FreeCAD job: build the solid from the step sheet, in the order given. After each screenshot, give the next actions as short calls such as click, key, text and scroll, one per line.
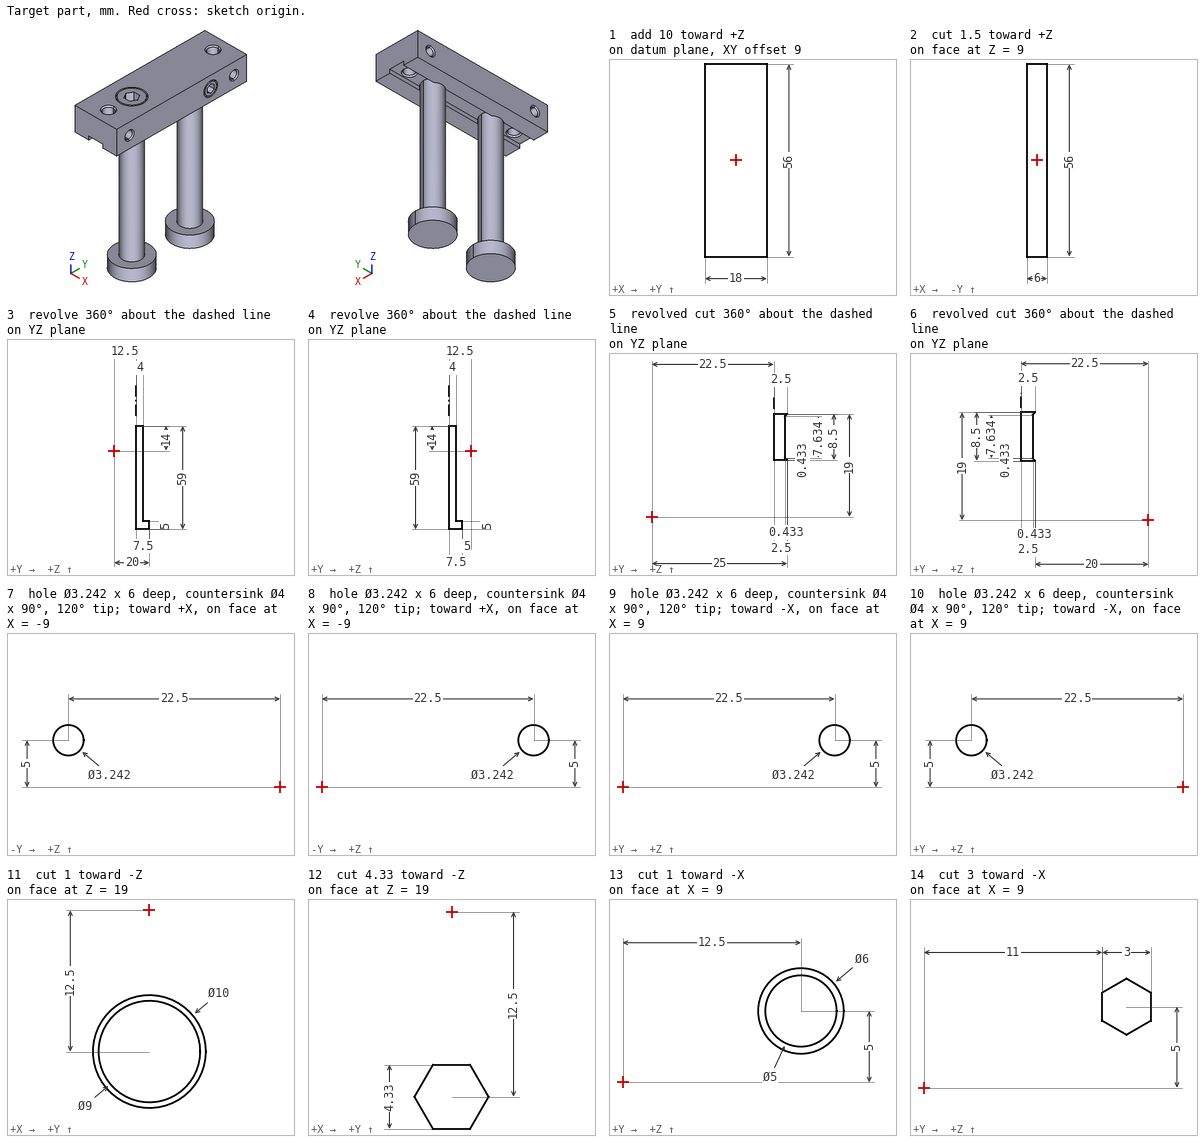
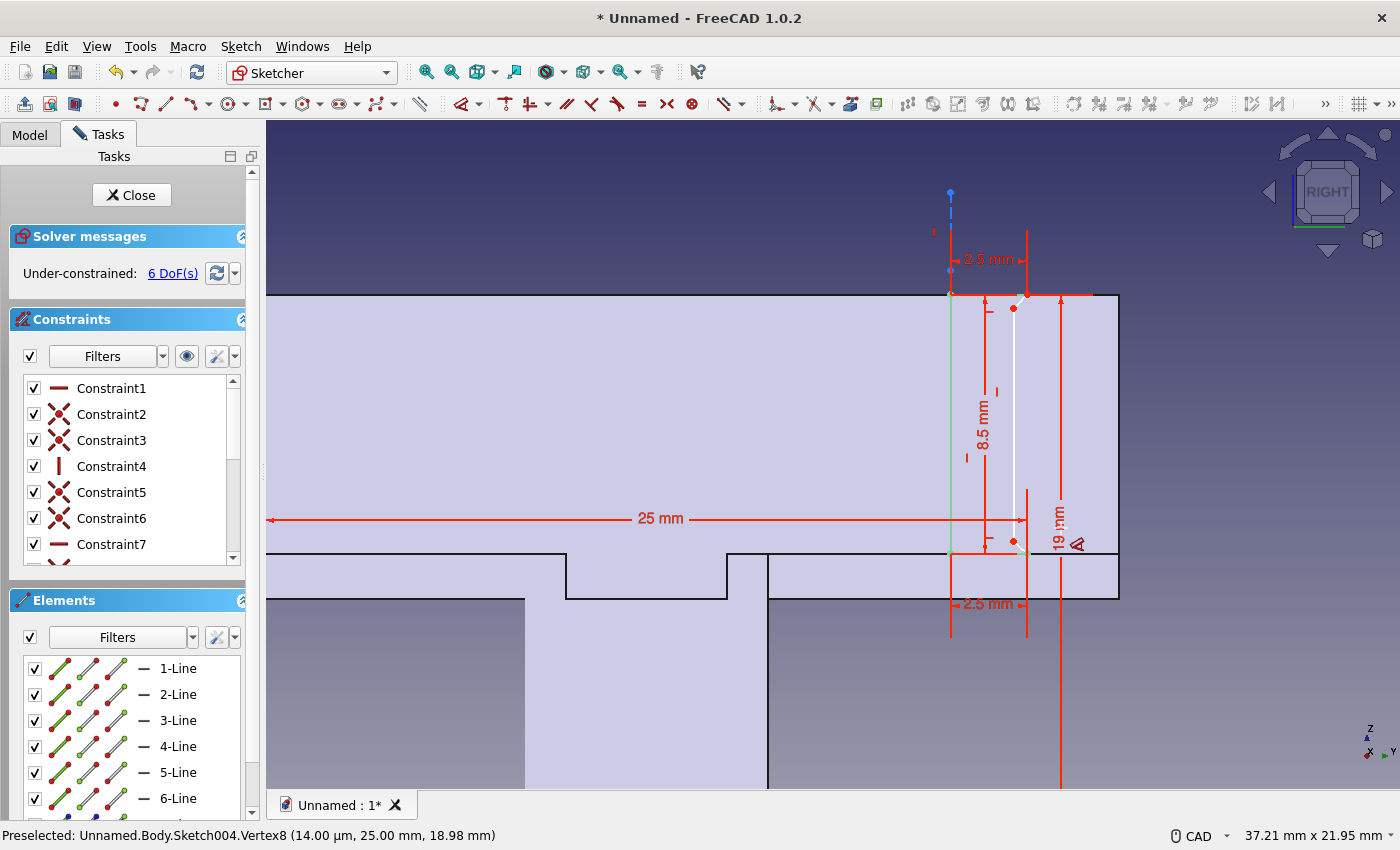
click(1014, 472)
click(1048, 371)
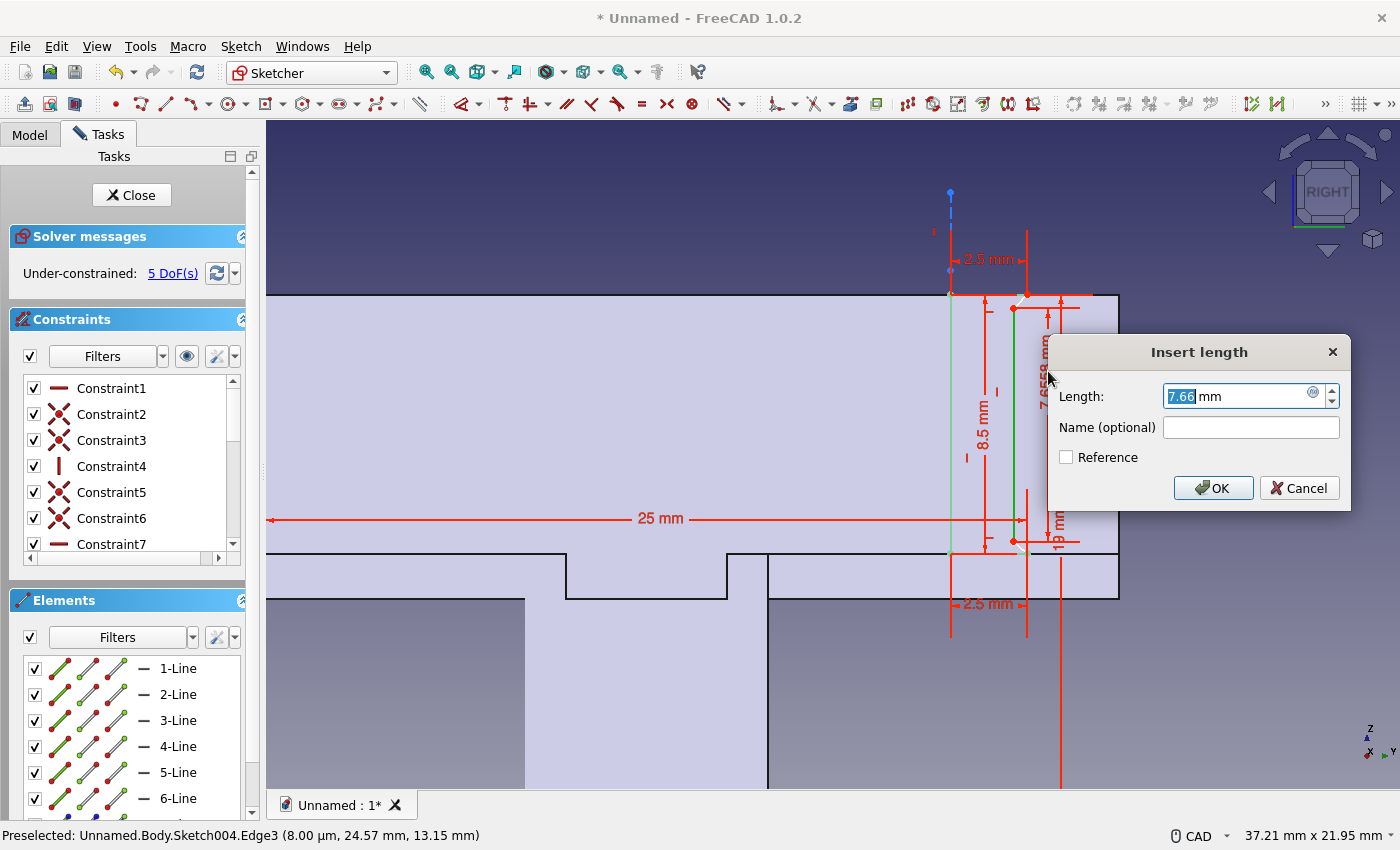
text(7.634)
key(Return)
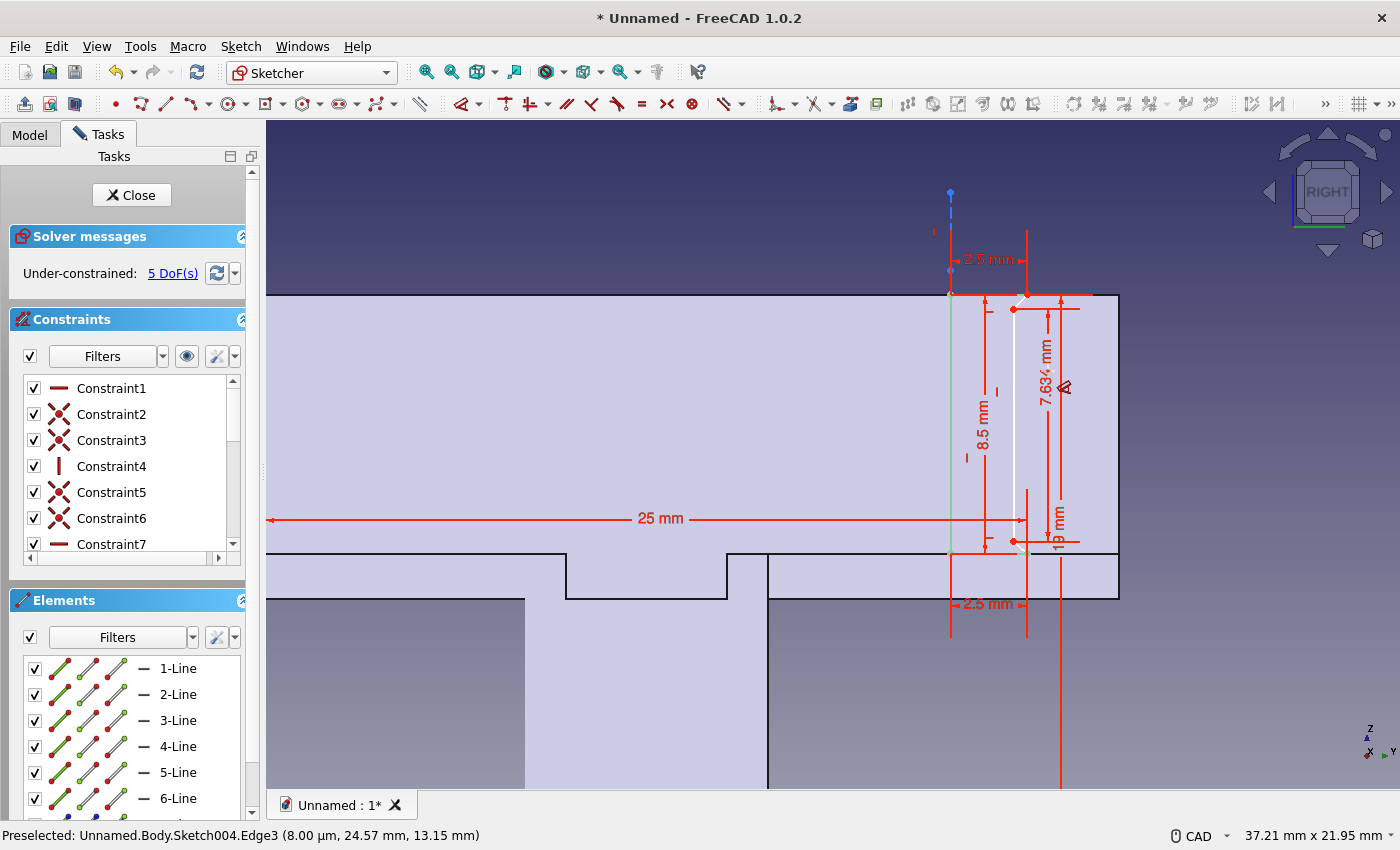
click(951, 271)
click(622, 237)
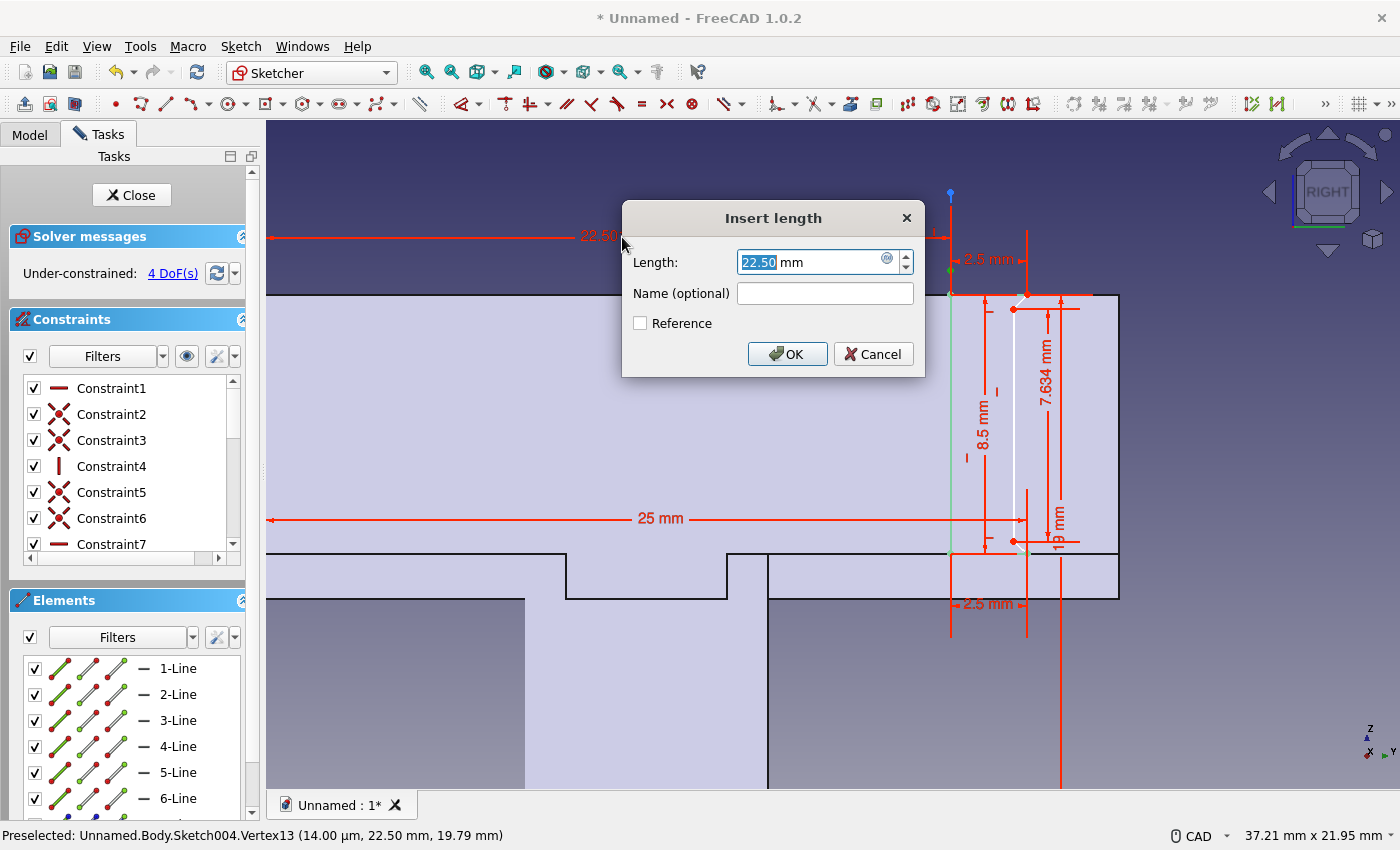
text(22.5)
key(Return)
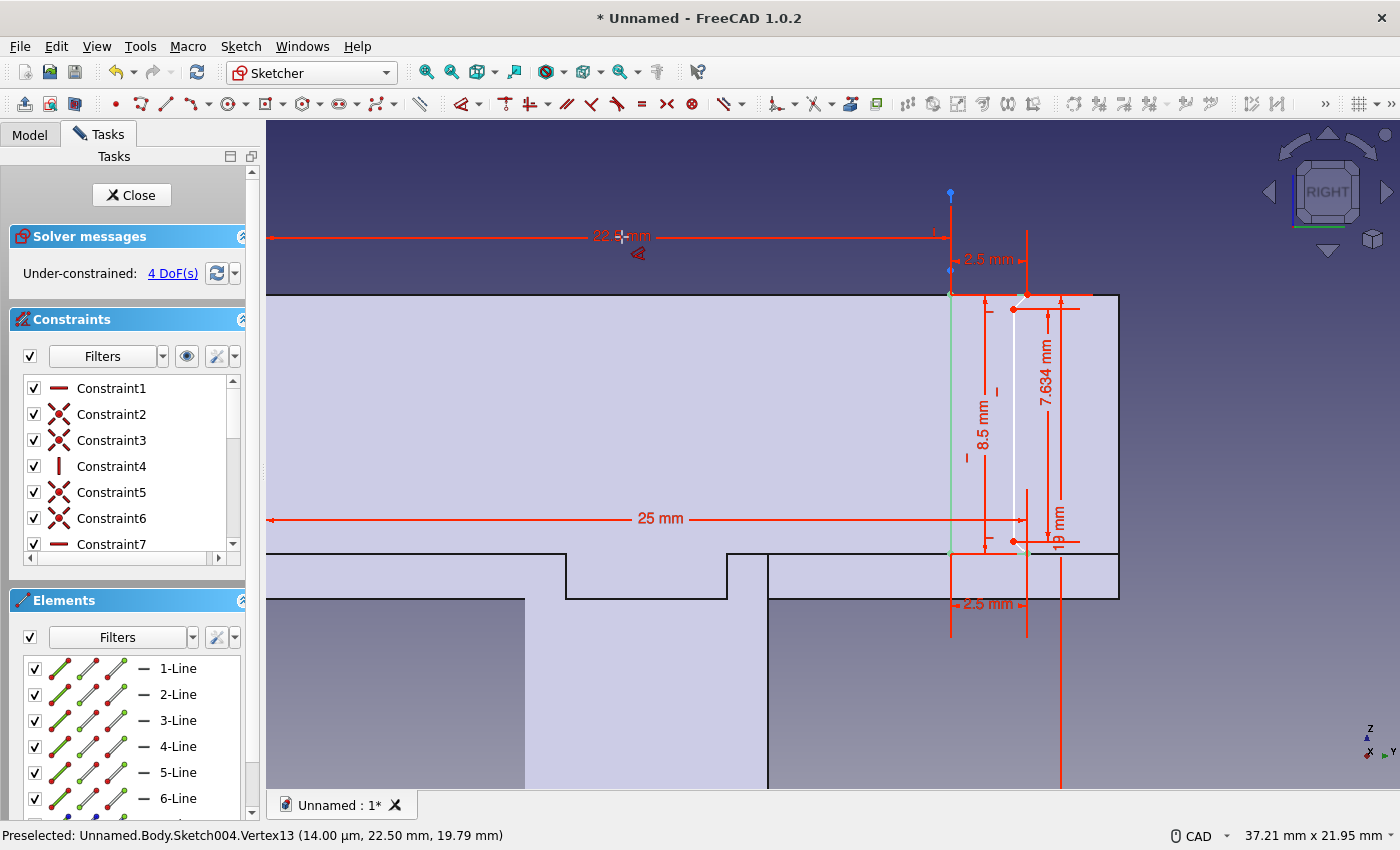
scroll(1019, 547, up, 6)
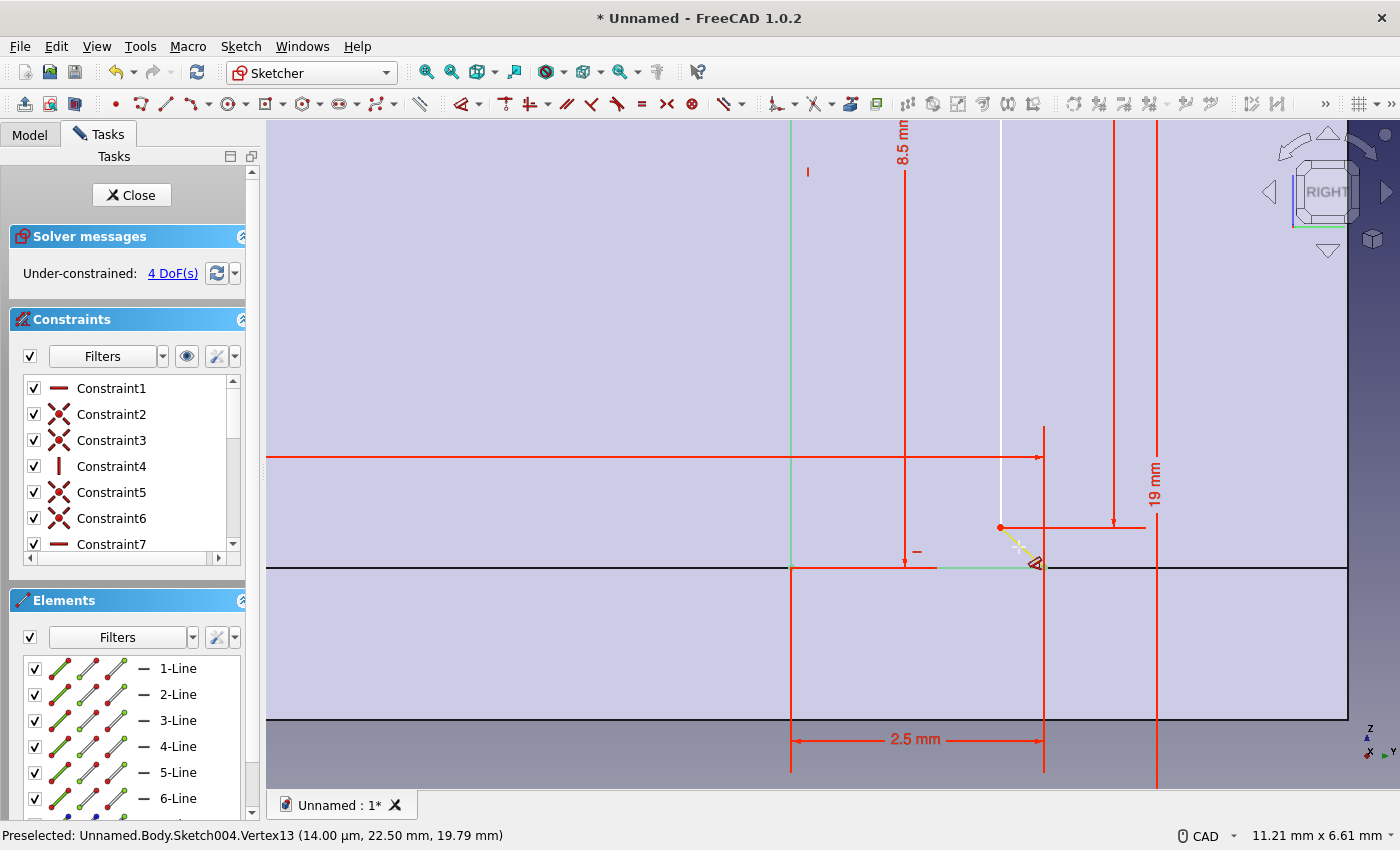
click(1018, 544)
click(1023, 602)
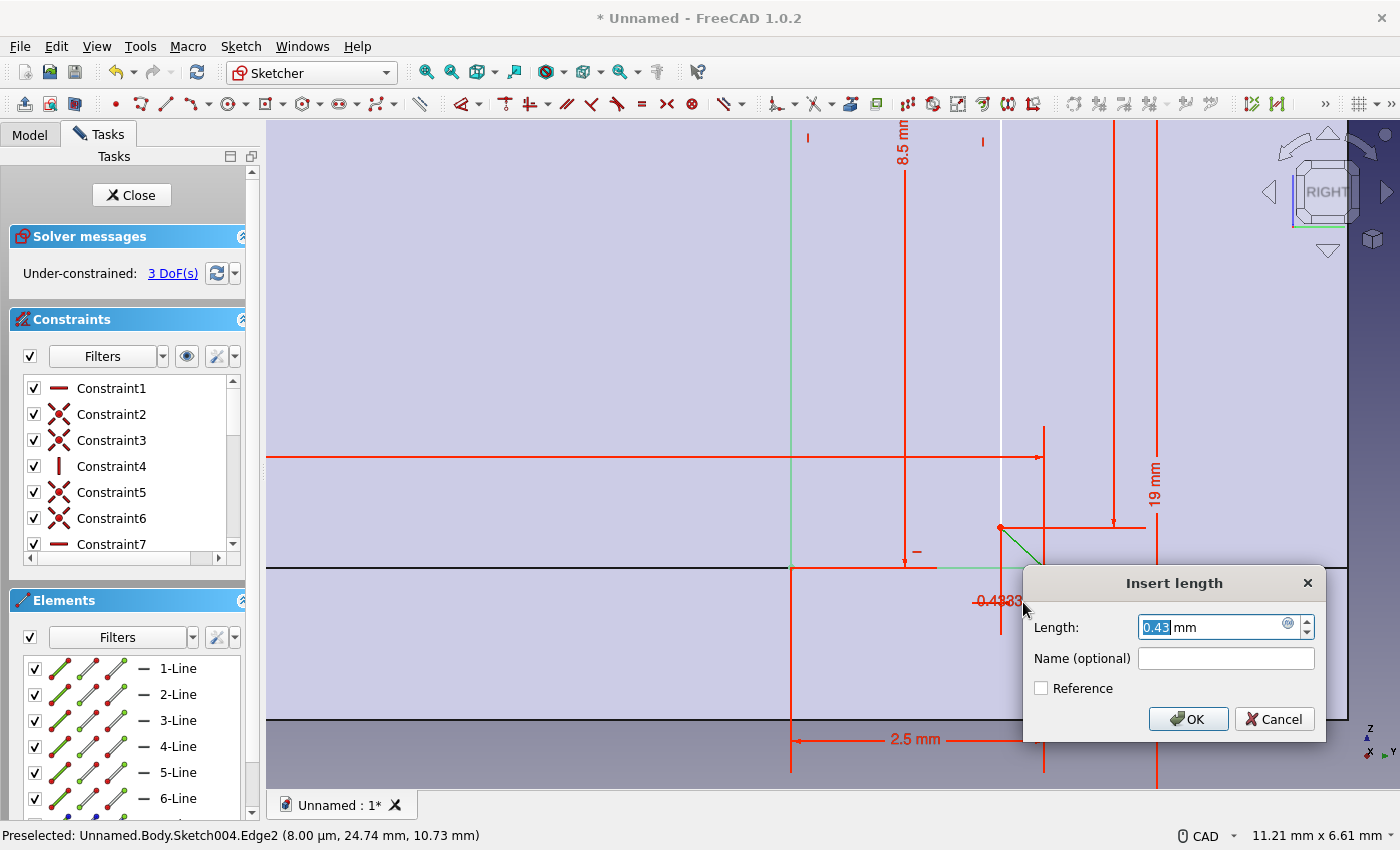
text(0.433)
key(Return)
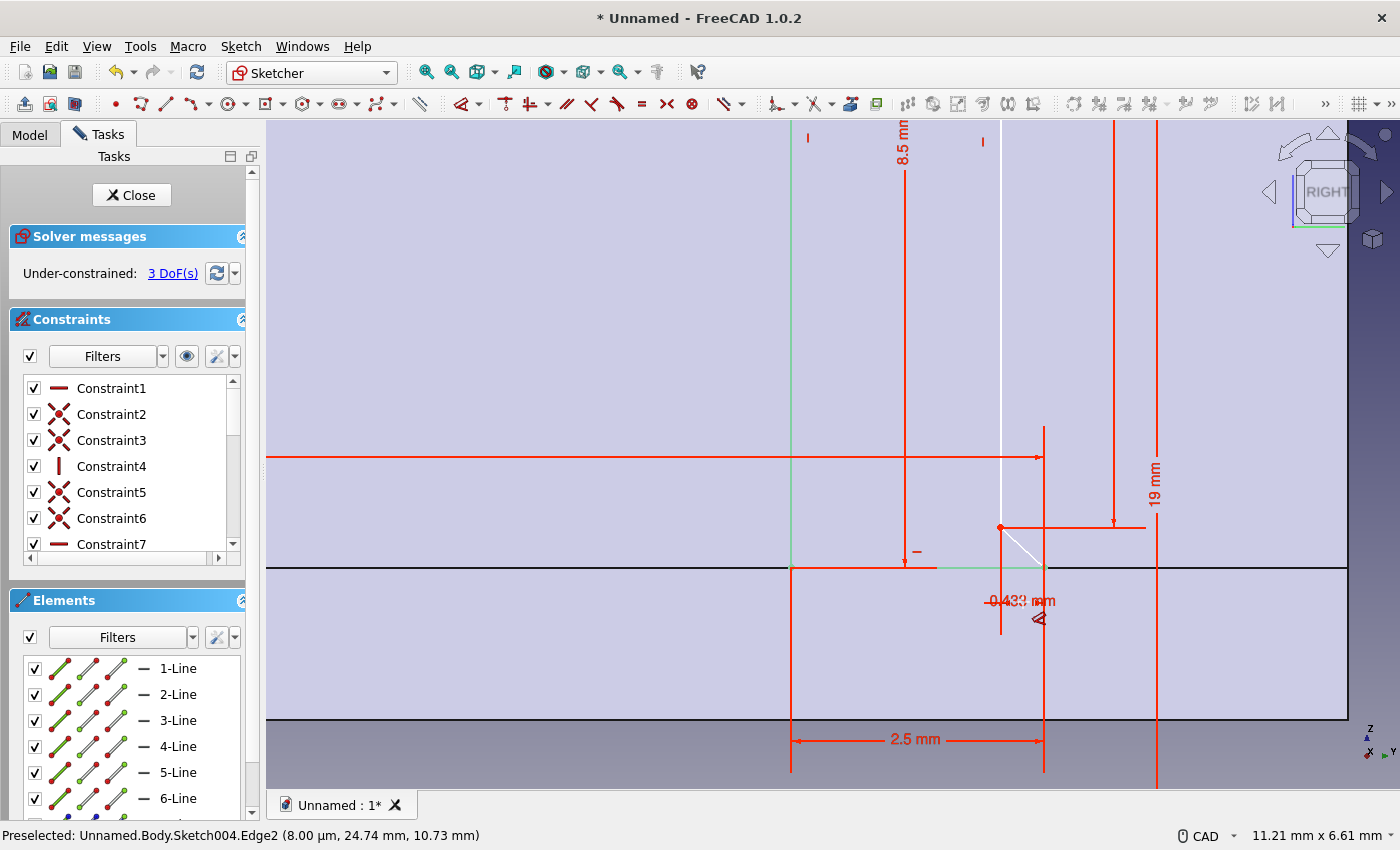
click(1031, 556)
click(1078, 548)